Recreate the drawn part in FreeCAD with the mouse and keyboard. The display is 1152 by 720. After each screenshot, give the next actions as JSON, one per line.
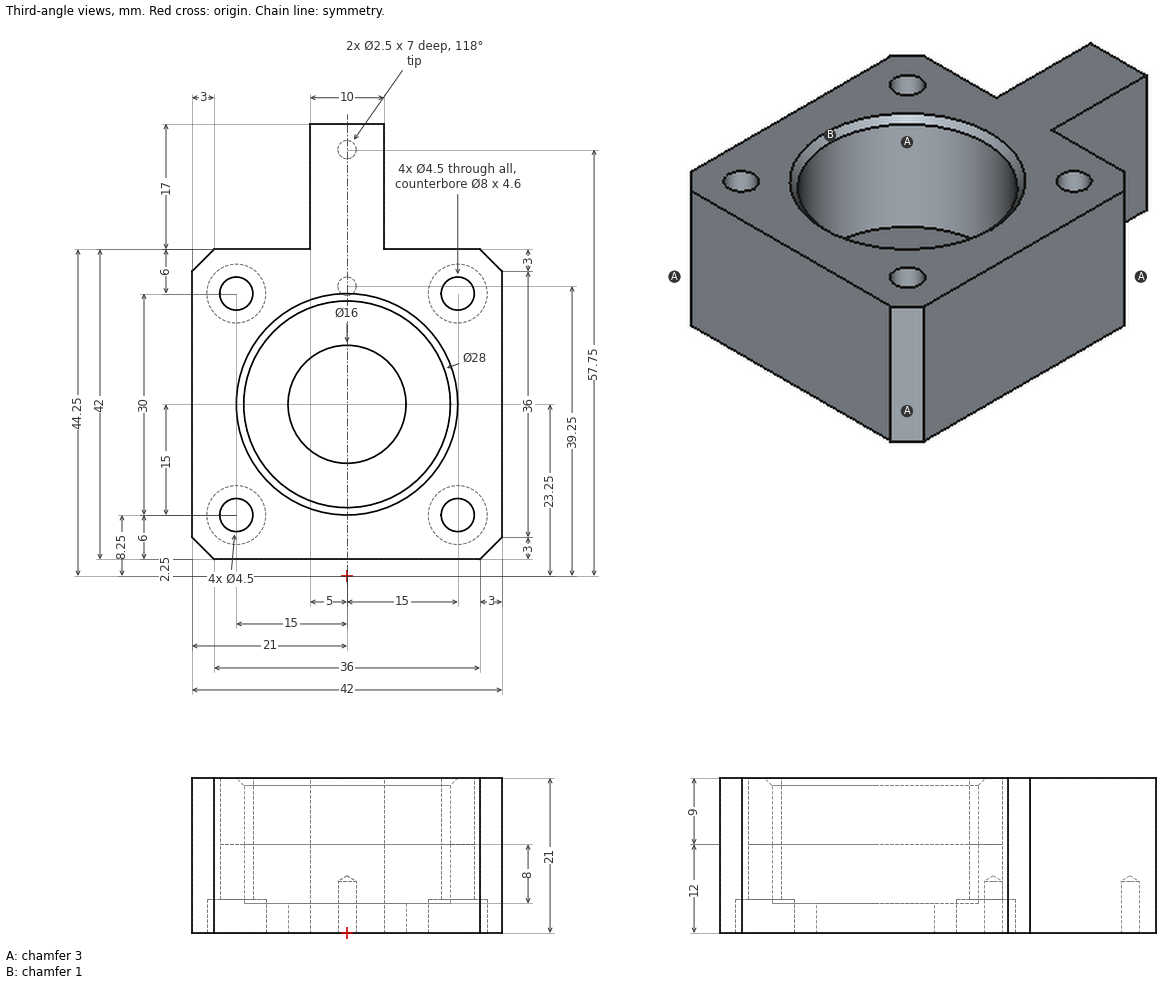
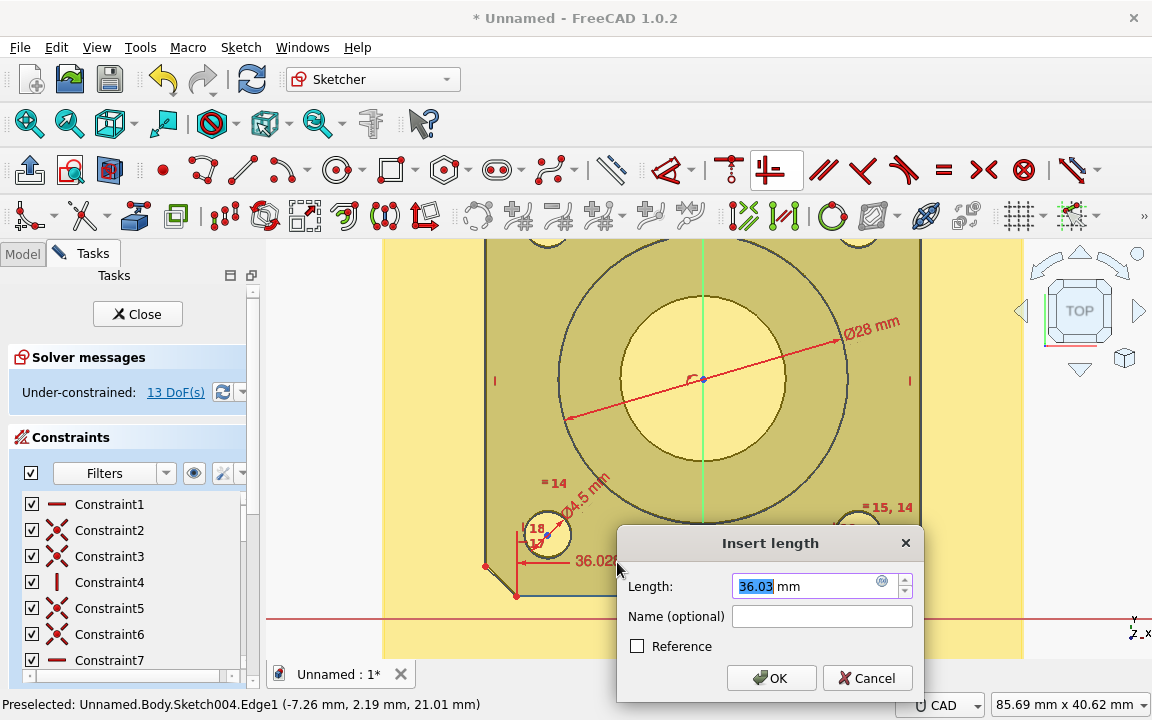
{"action": "type", "text": "36"}
{"action": "key", "text": "Return"}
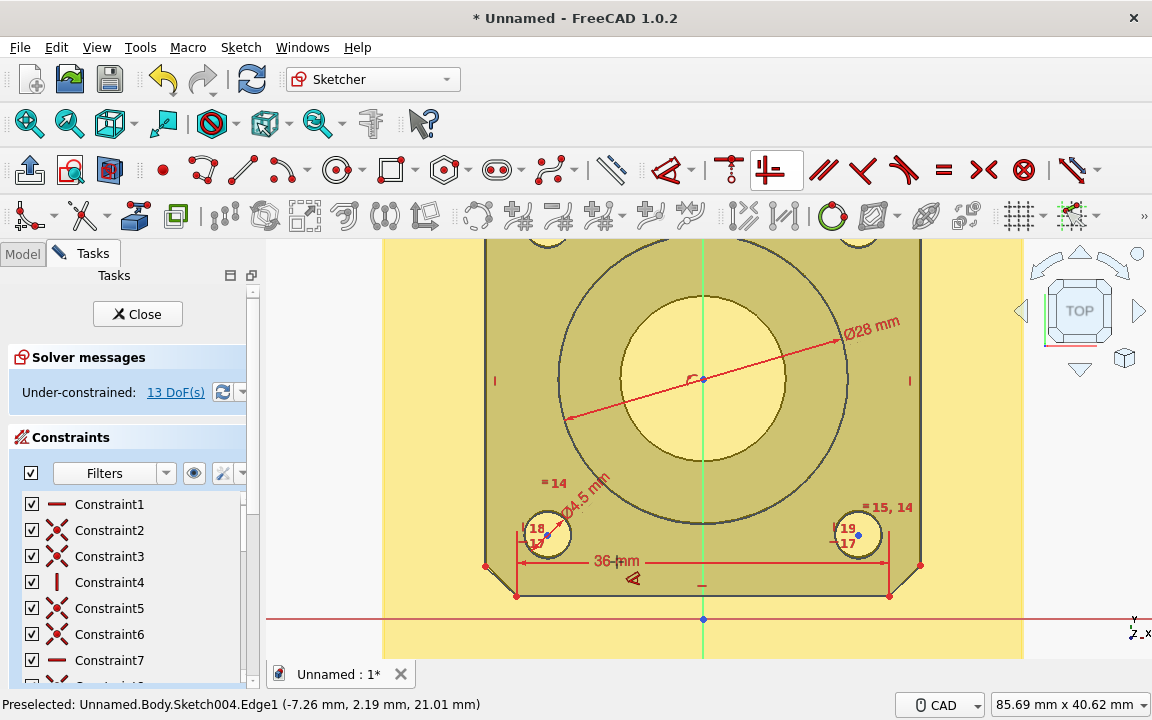
{"action": "left_click", "coordinate": [921, 455]}
{"action": "left_click", "coordinate": [955, 416]}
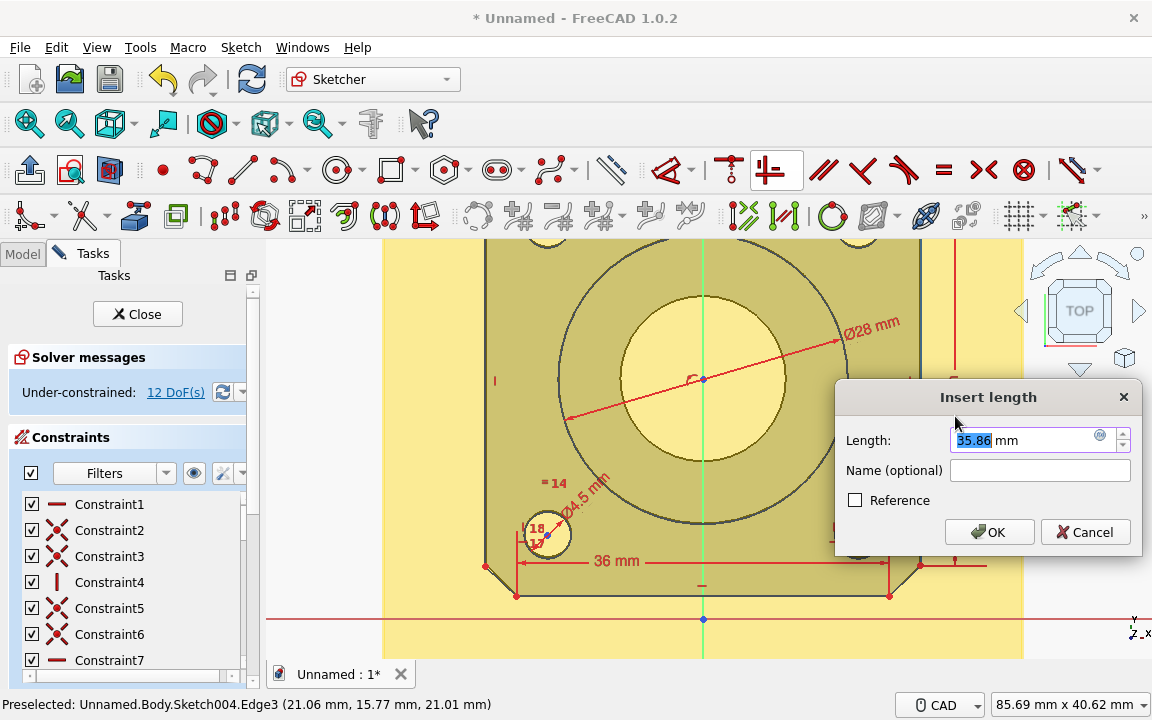
{"action": "type", "text": "36"}
{"action": "key", "text": "Return"}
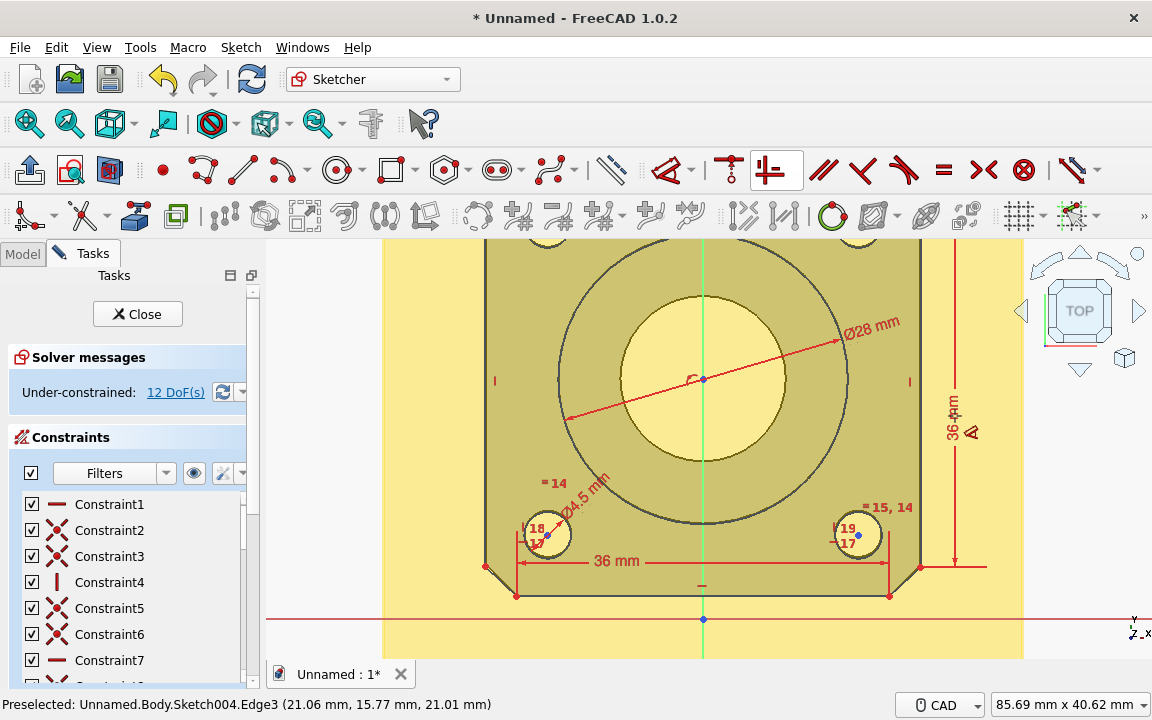
{"action": "scroll", "coordinate": [564, 520], "scroll_direction": "down", "scroll_amount": 3}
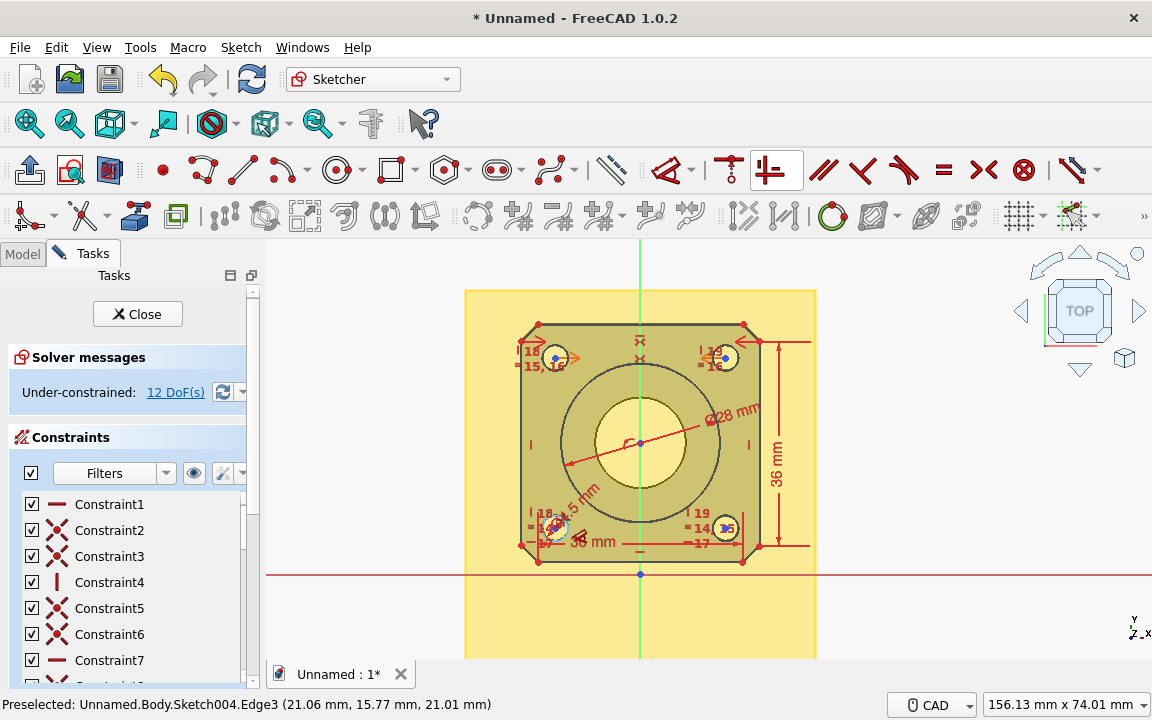
{"action": "left_click", "coordinate": [682, 325]}
{"action": "left_click", "coordinate": [593, 291]}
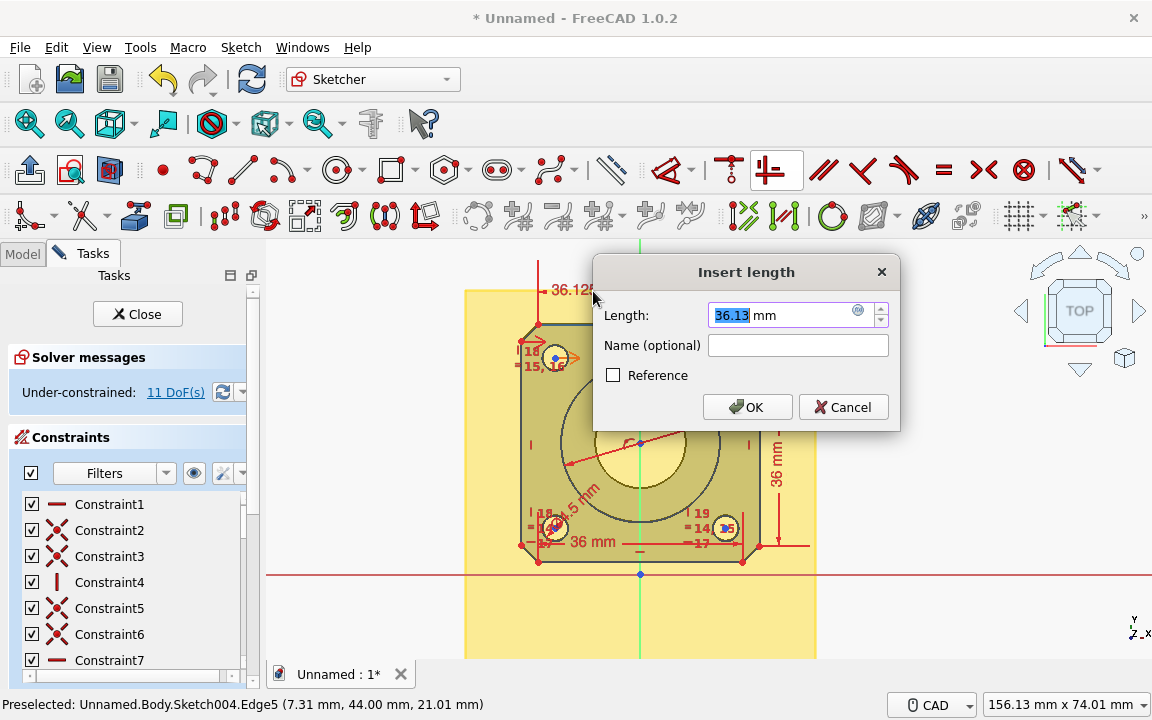
{"action": "type", "text": "36"}
{"action": "key", "text": "Return"}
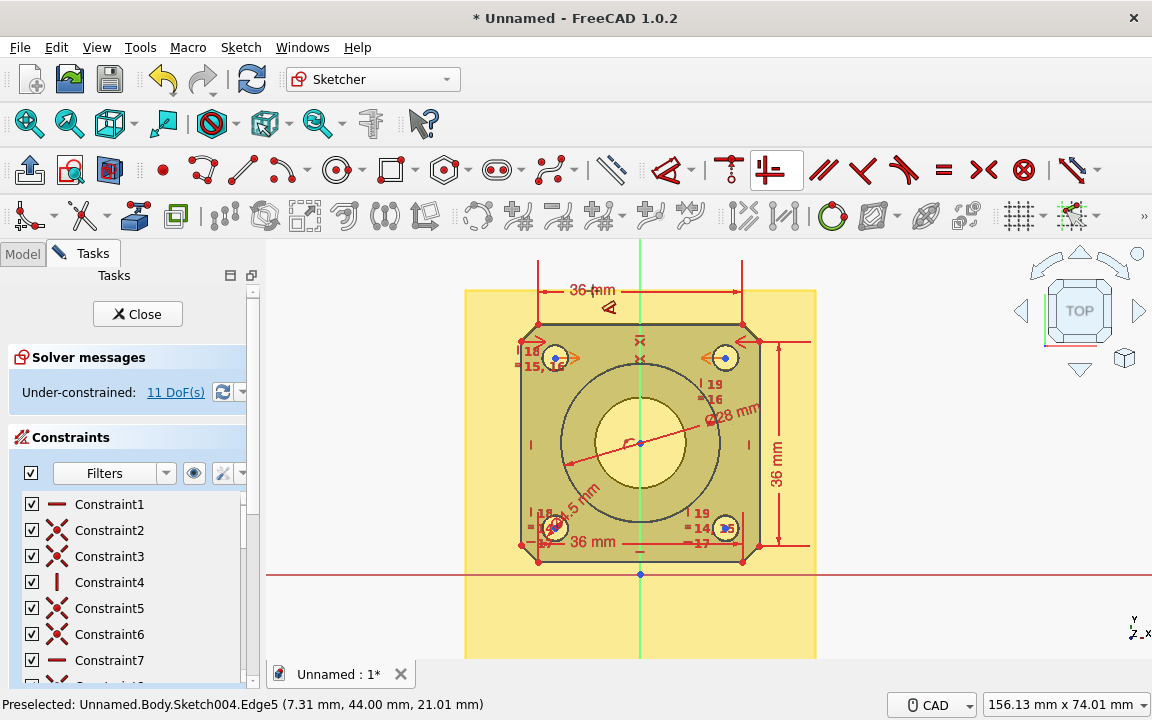
{"action": "left_click", "coordinate": [521, 403]}
{"action": "left_click", "coordinate": [487, 444]}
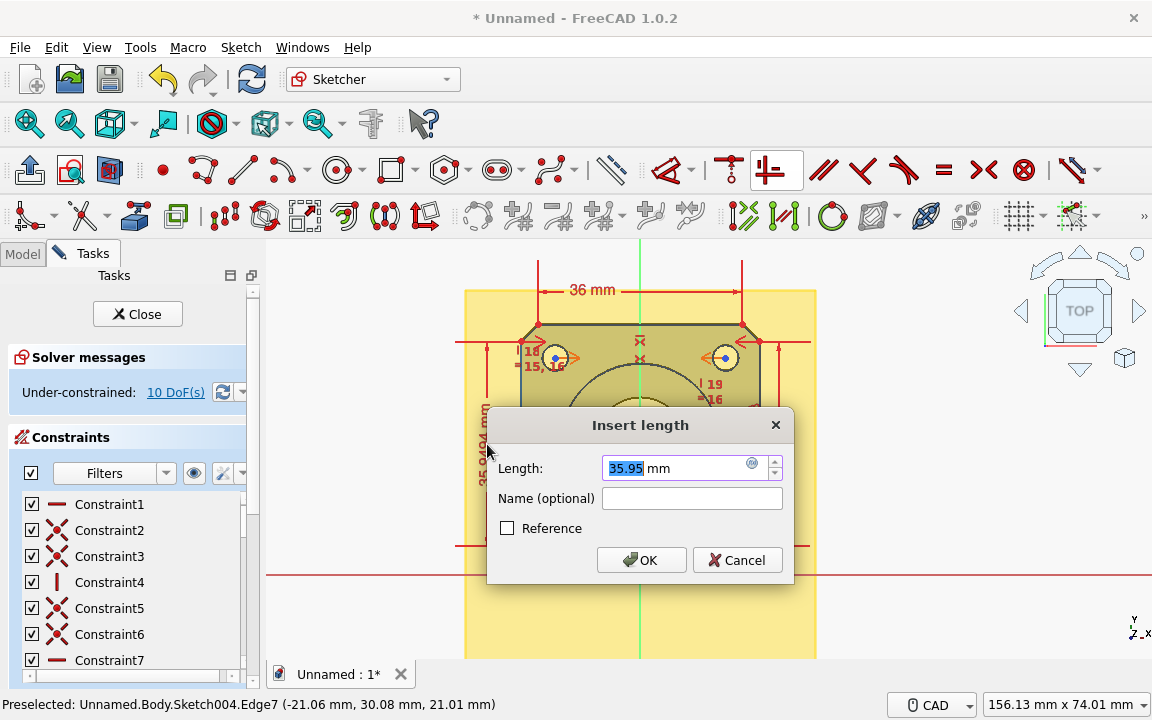
{"action": "type", "text": "36"}
{"action": "key", "text": "Return"}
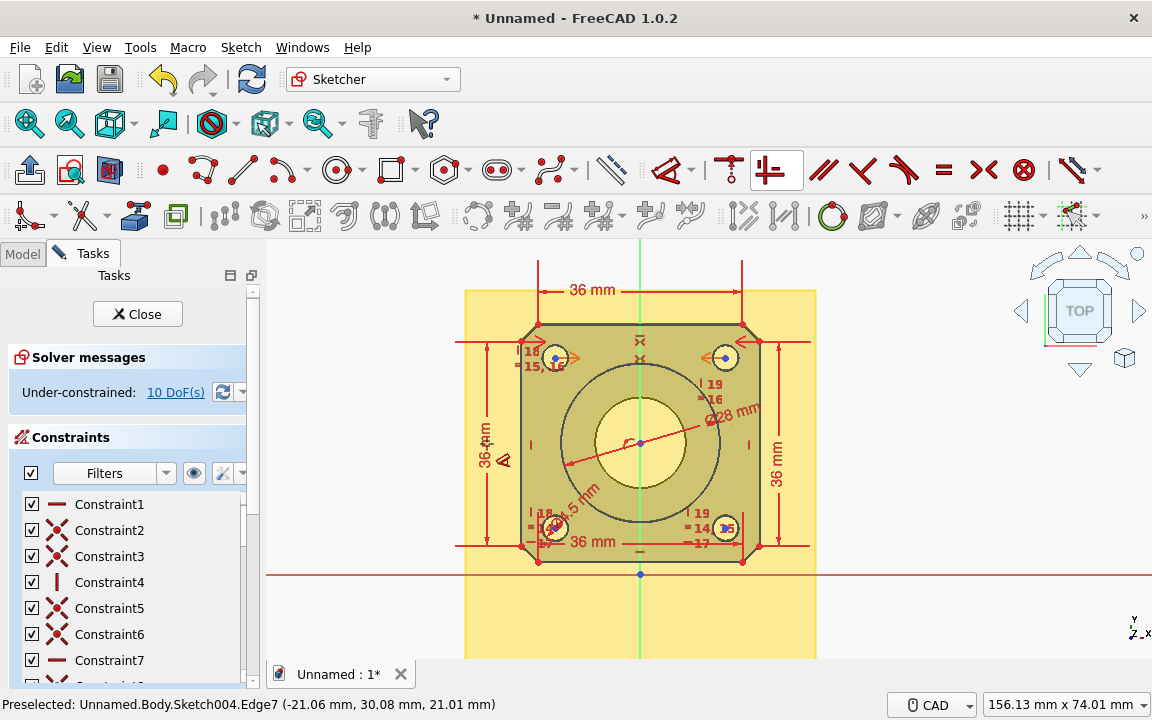
{"action": "scroll", "coordinate": [750, 556], "scroll_direction": "up", "scroll_amount": 5}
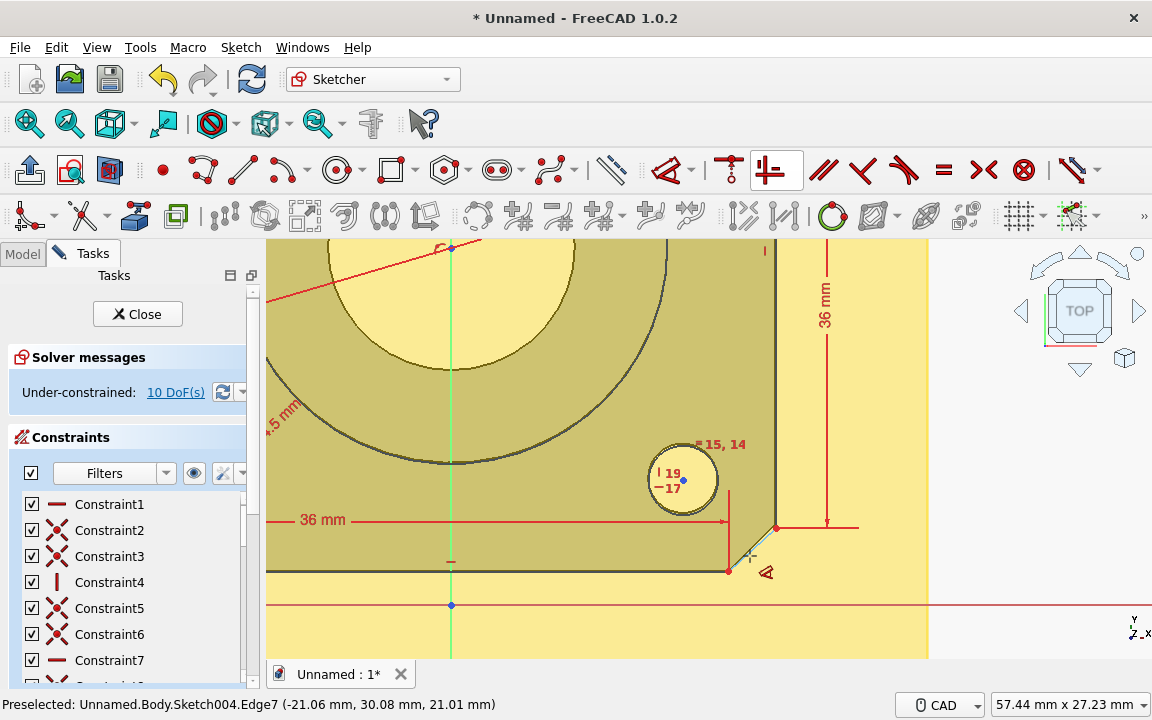
{"action": "left_click", "coordinate": [748, 554]}
{"action": "left_click", "coordinate": [752, 494]}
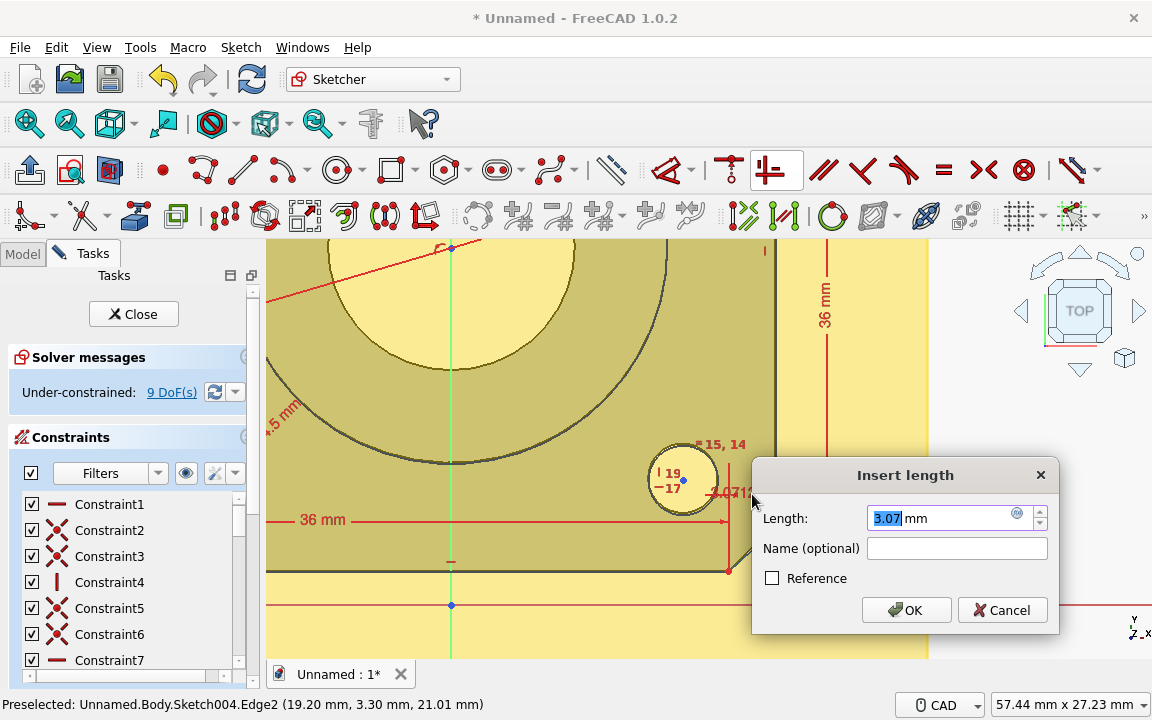
{"action": "type", "text": "3"}
{"action": "key", "text": "Return"}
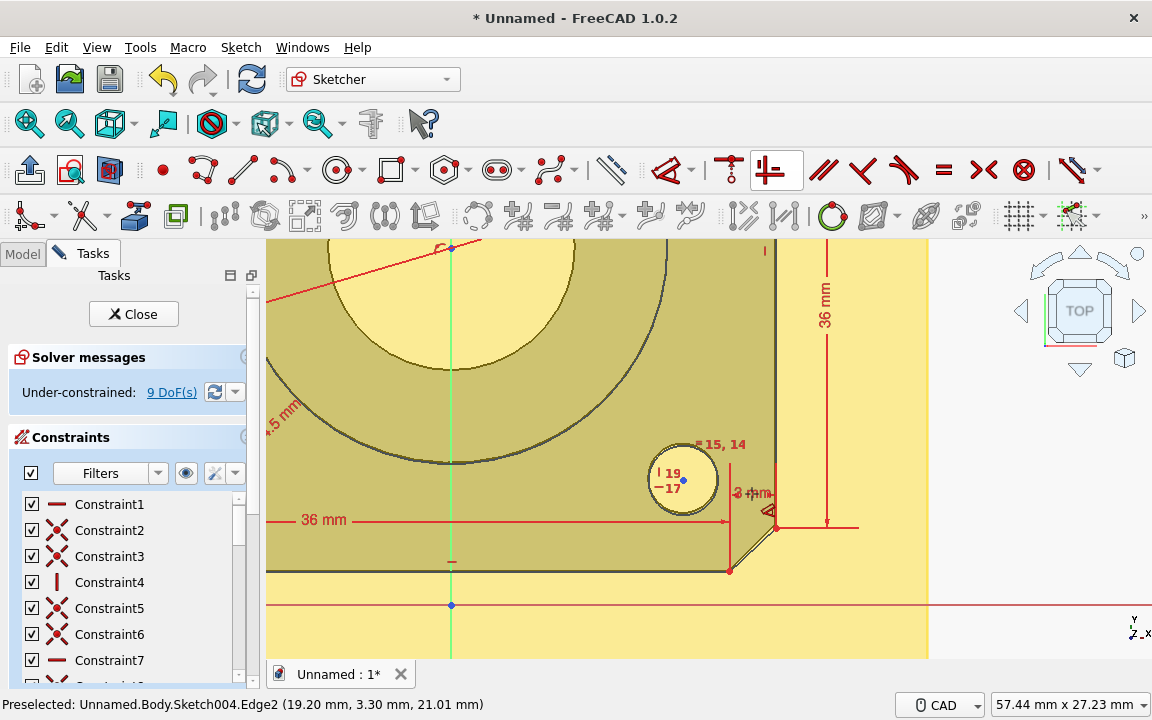
{"action": "left_click", "coordinate": [744, 559]}
{"action": "left_click", "coordinate": [810, 550]}